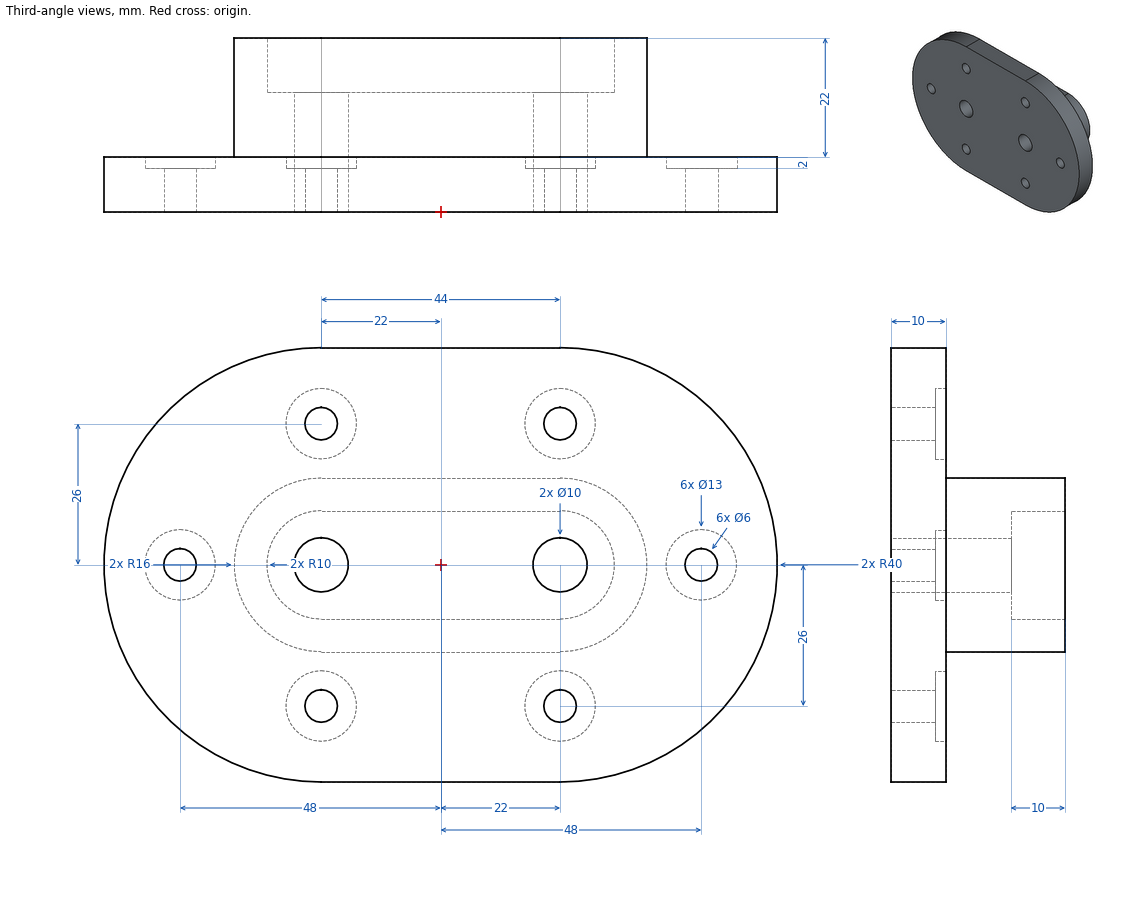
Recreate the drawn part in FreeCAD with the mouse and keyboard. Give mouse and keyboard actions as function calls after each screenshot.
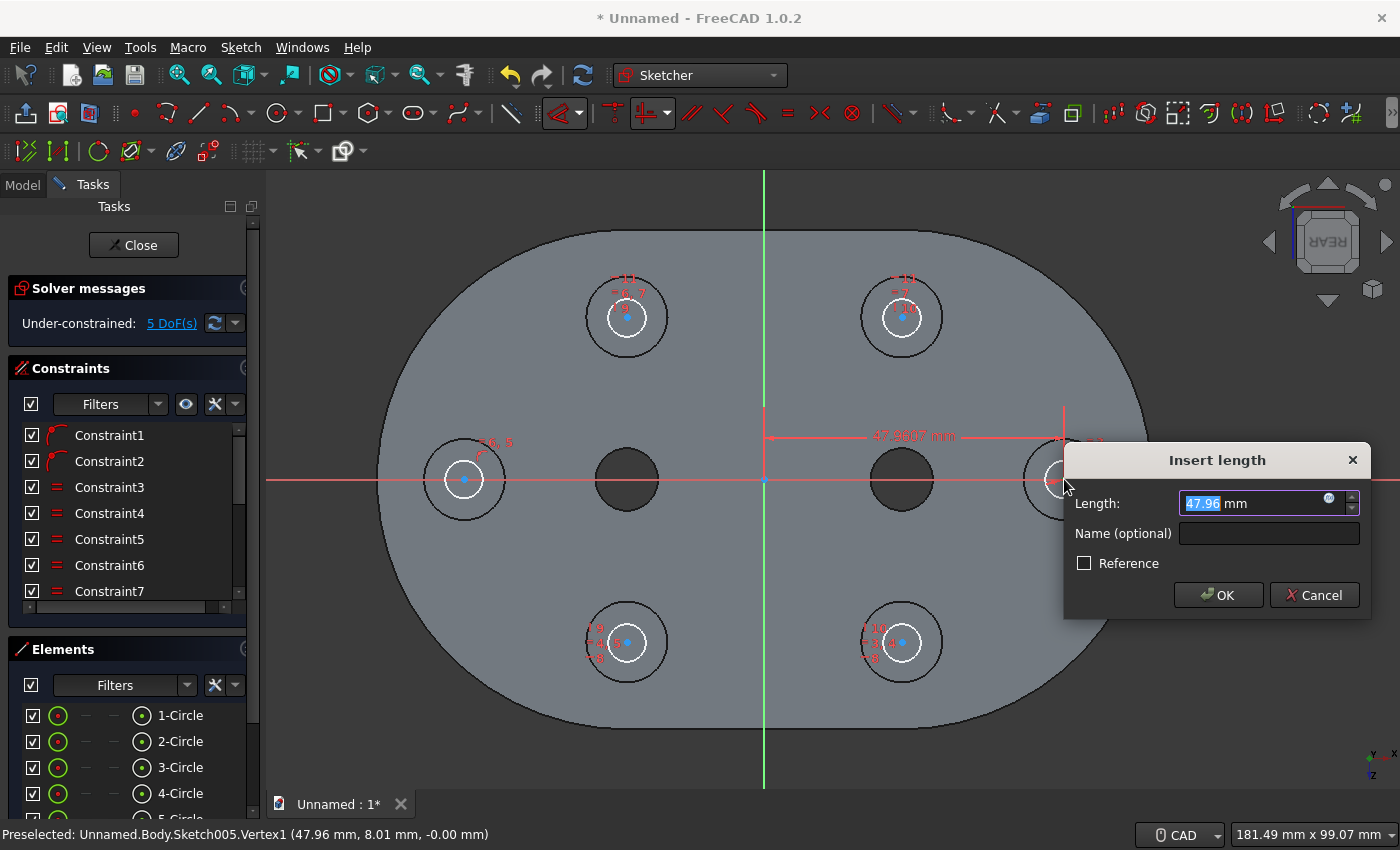
text(48)
key(Return)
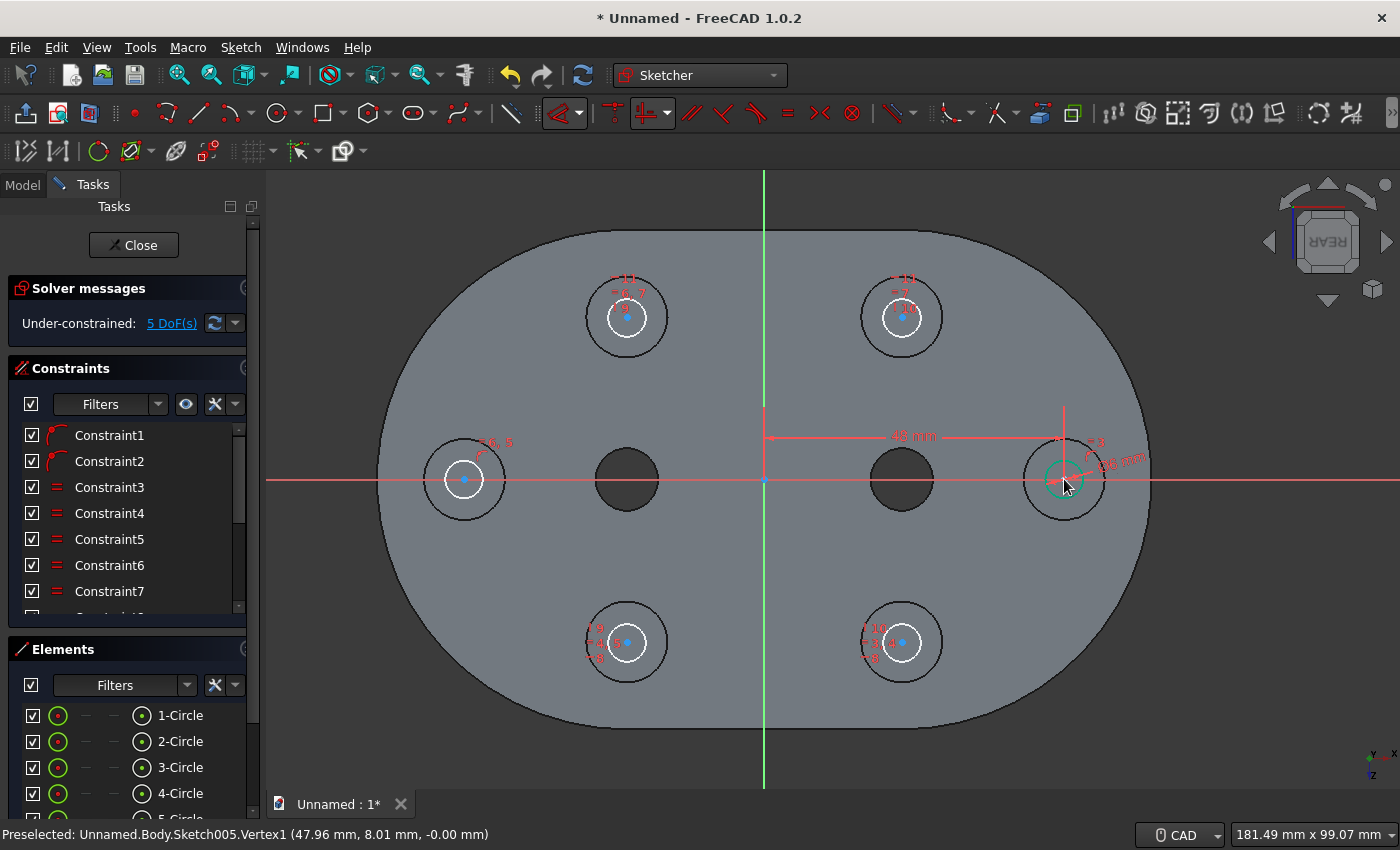
click(902, 643)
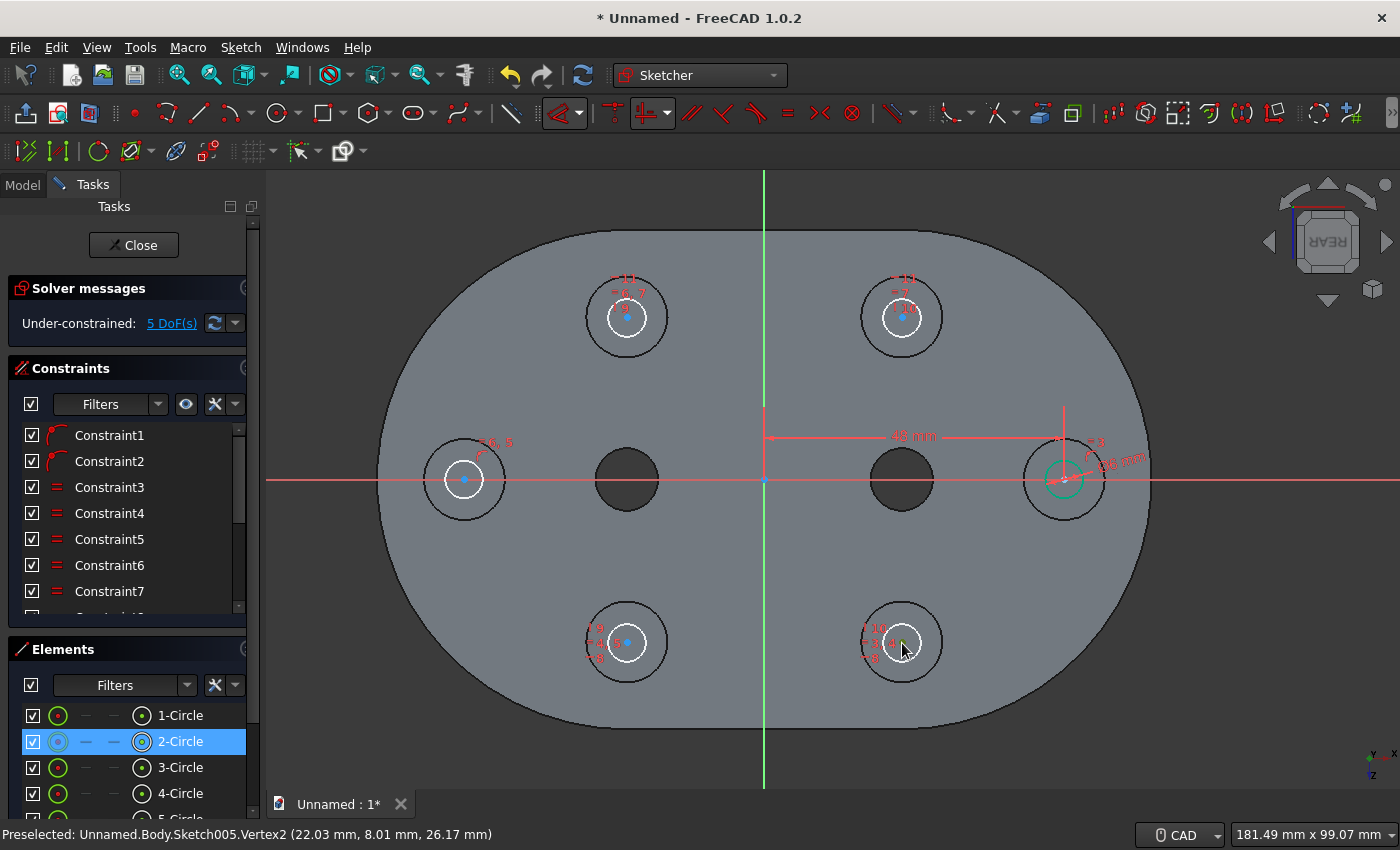
click(582, 114)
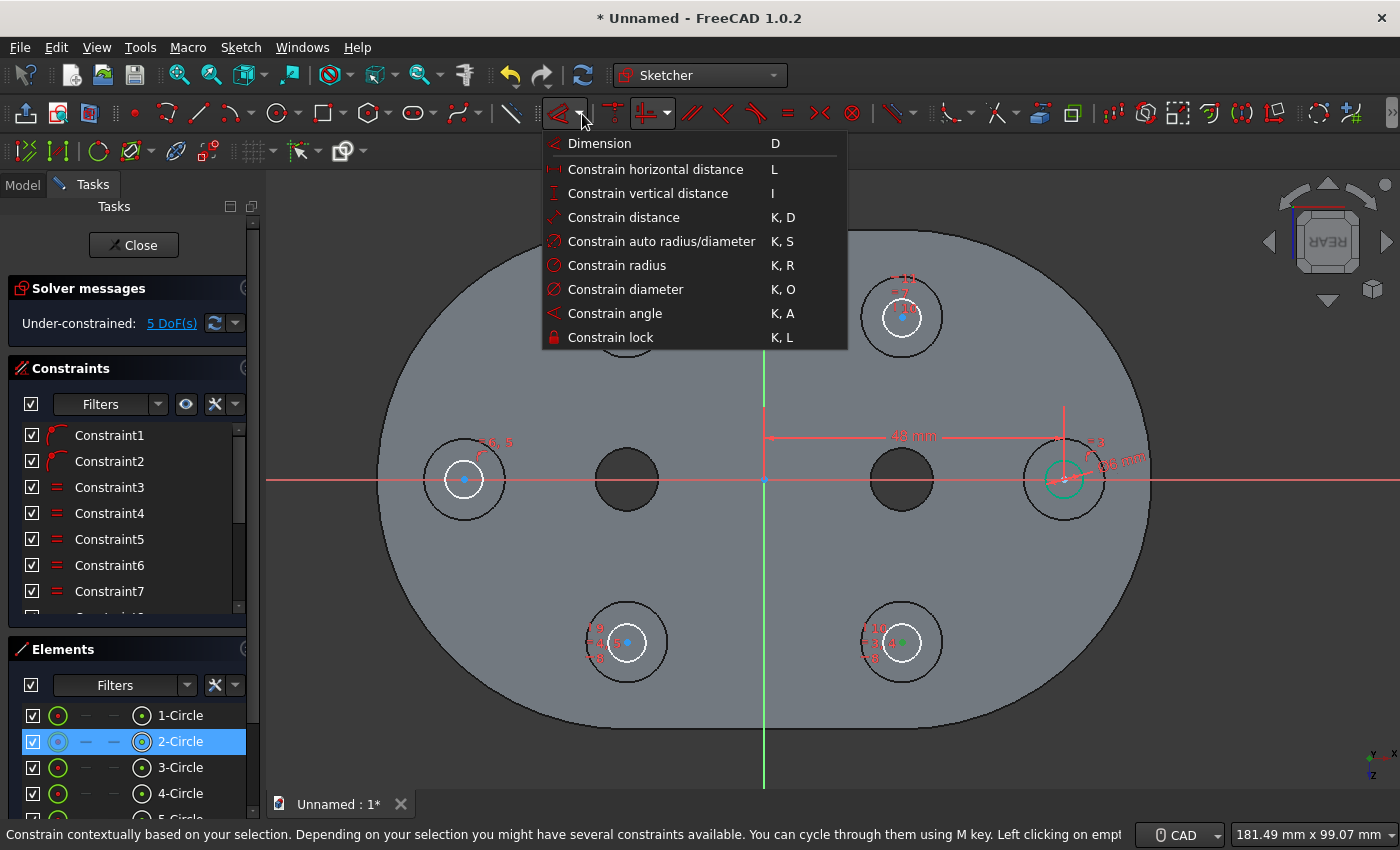
click(695, 169)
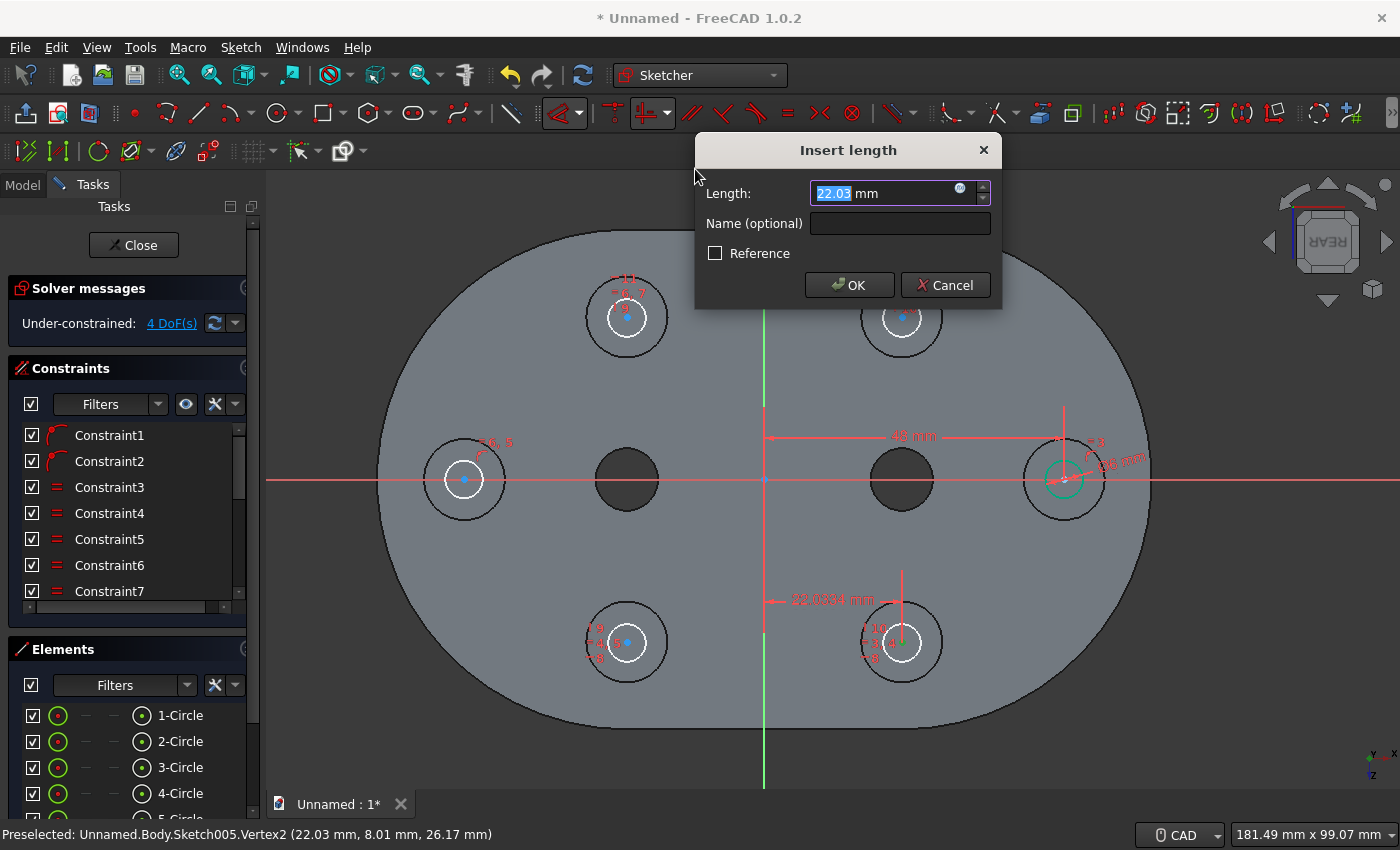
text(22)
key(Return)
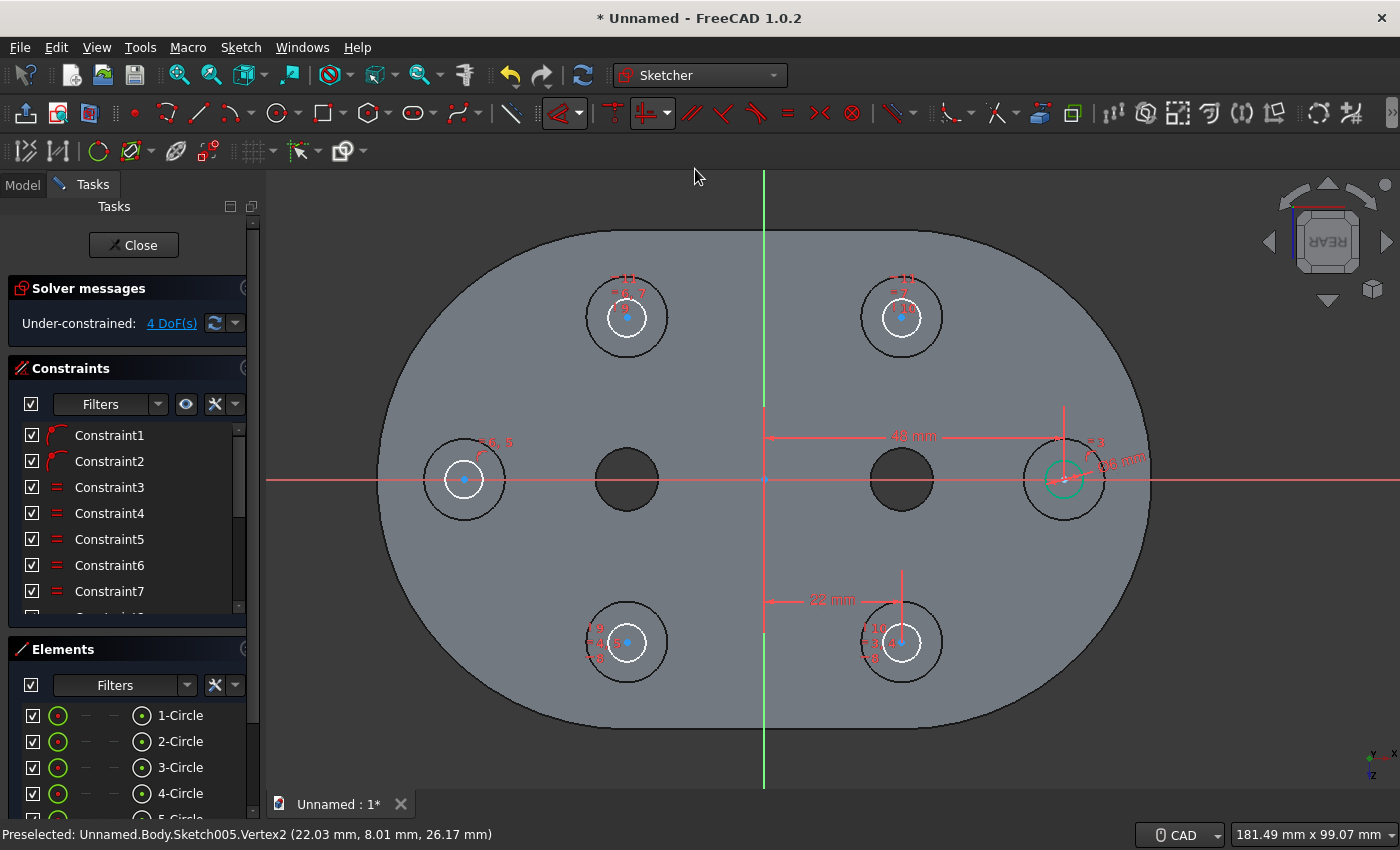
click(902, 643)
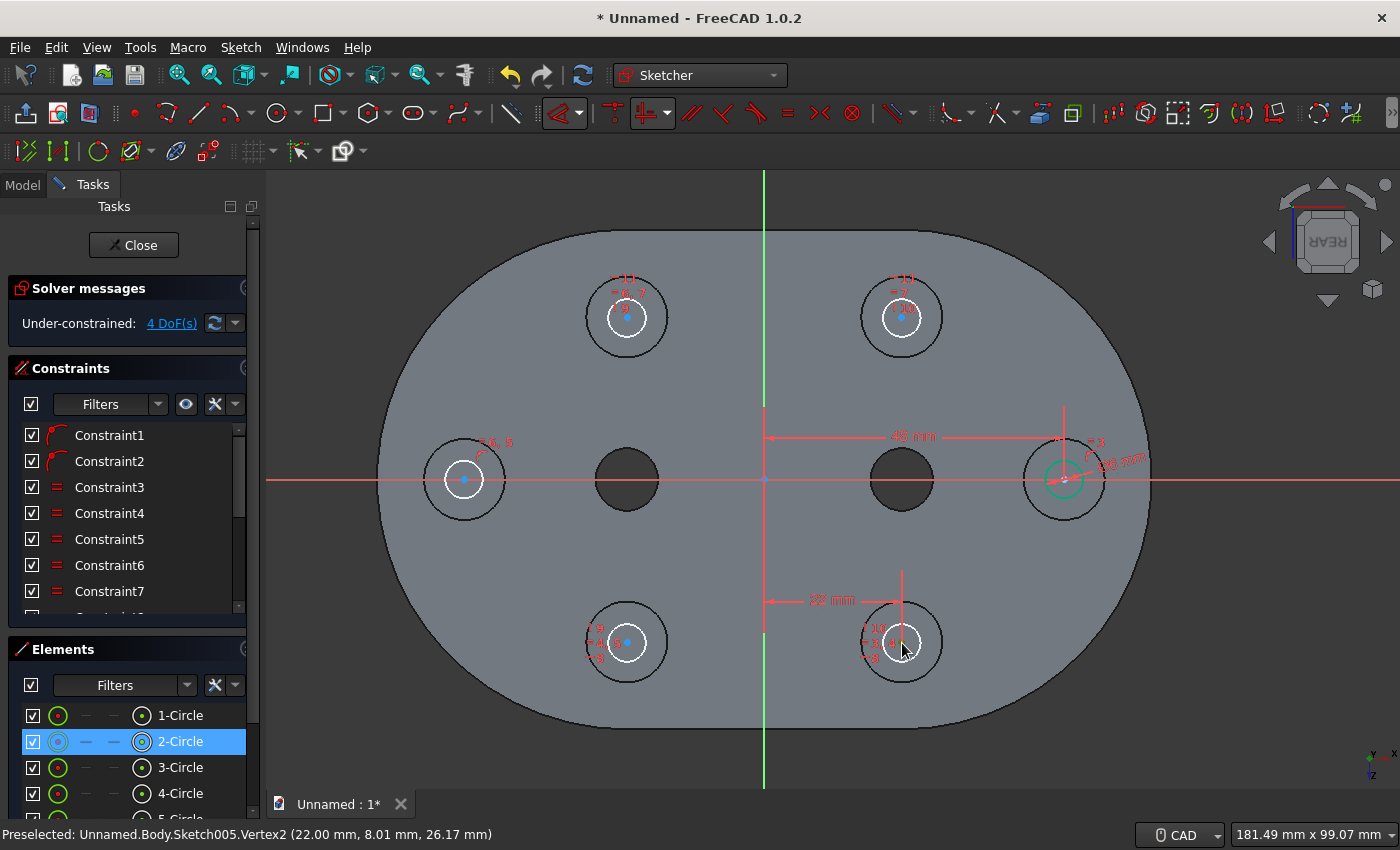
click(582, 114)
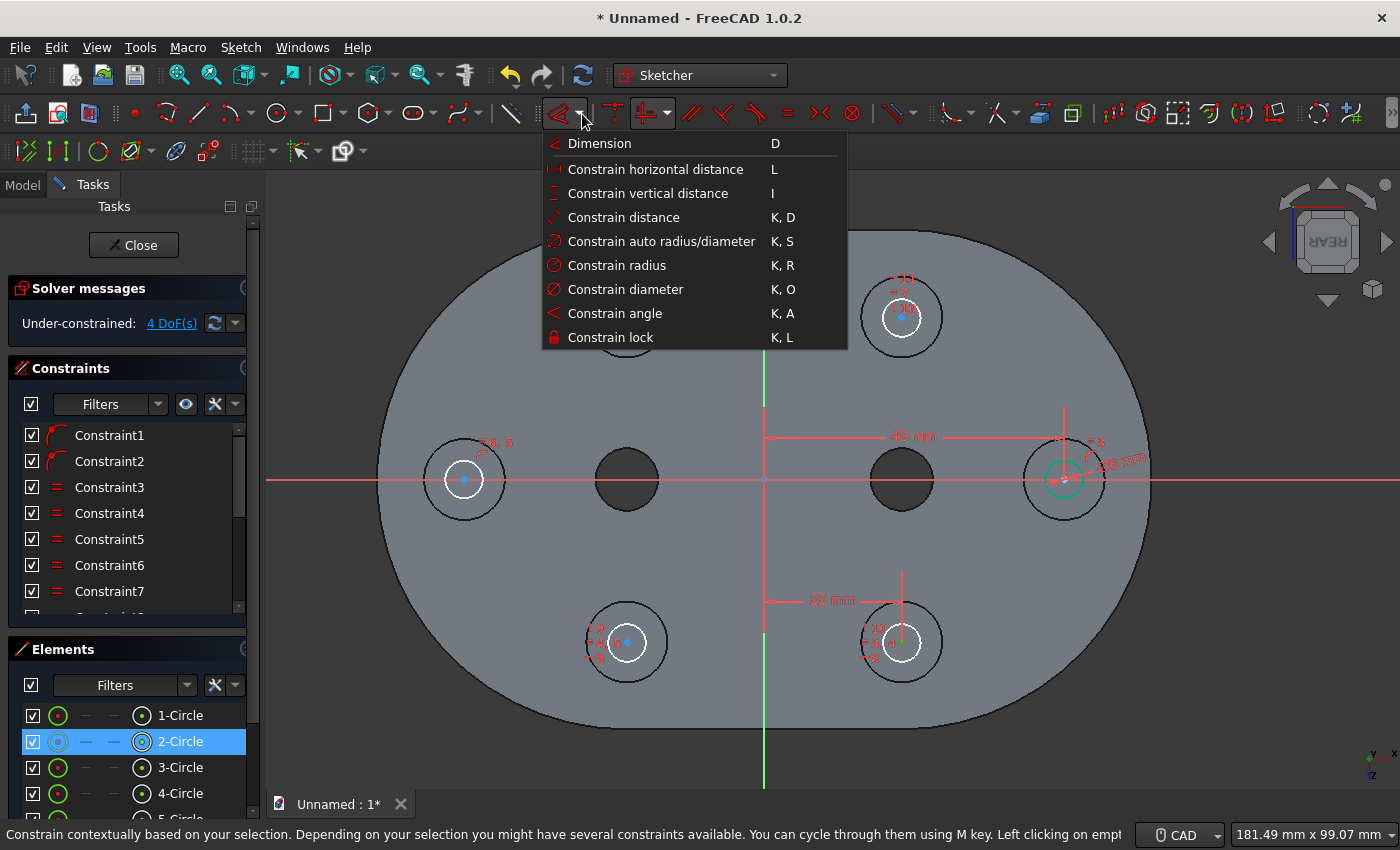
click(695, 193)